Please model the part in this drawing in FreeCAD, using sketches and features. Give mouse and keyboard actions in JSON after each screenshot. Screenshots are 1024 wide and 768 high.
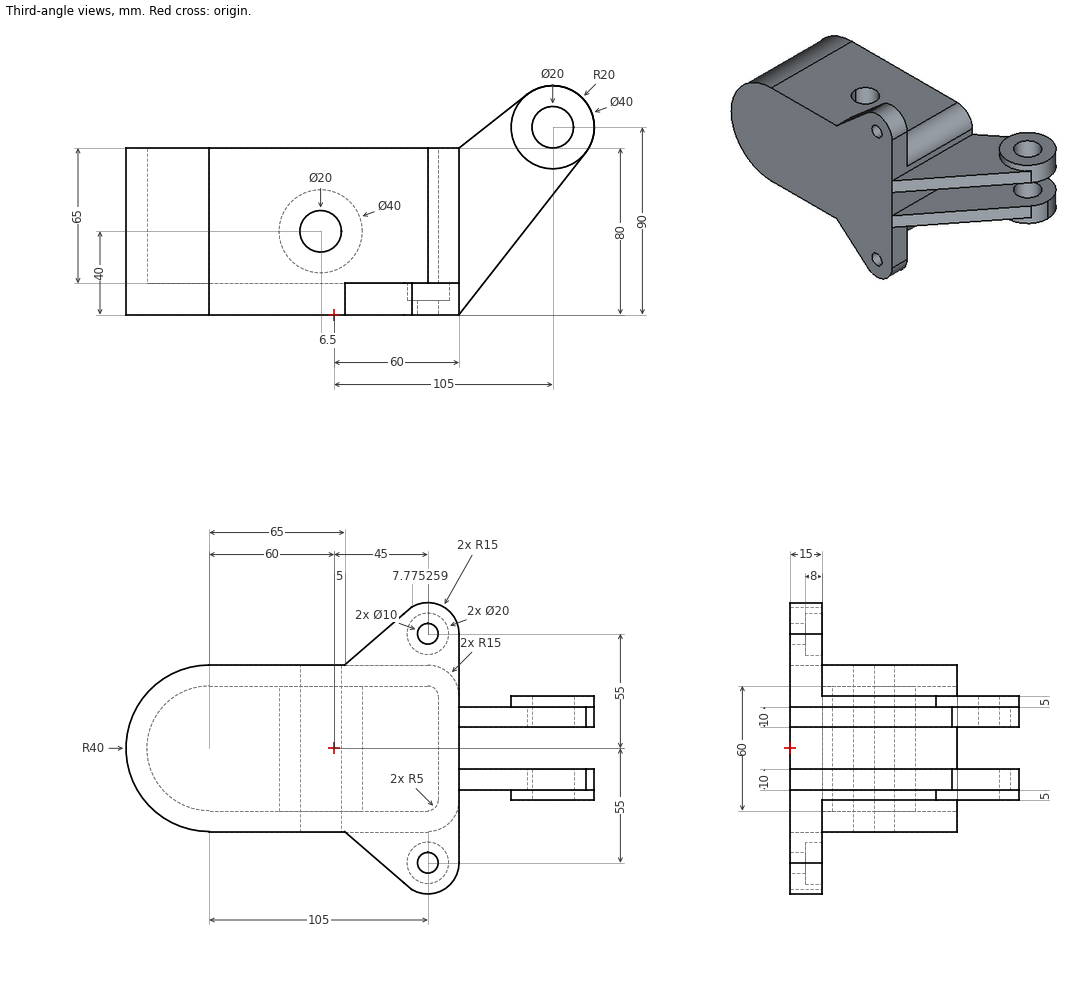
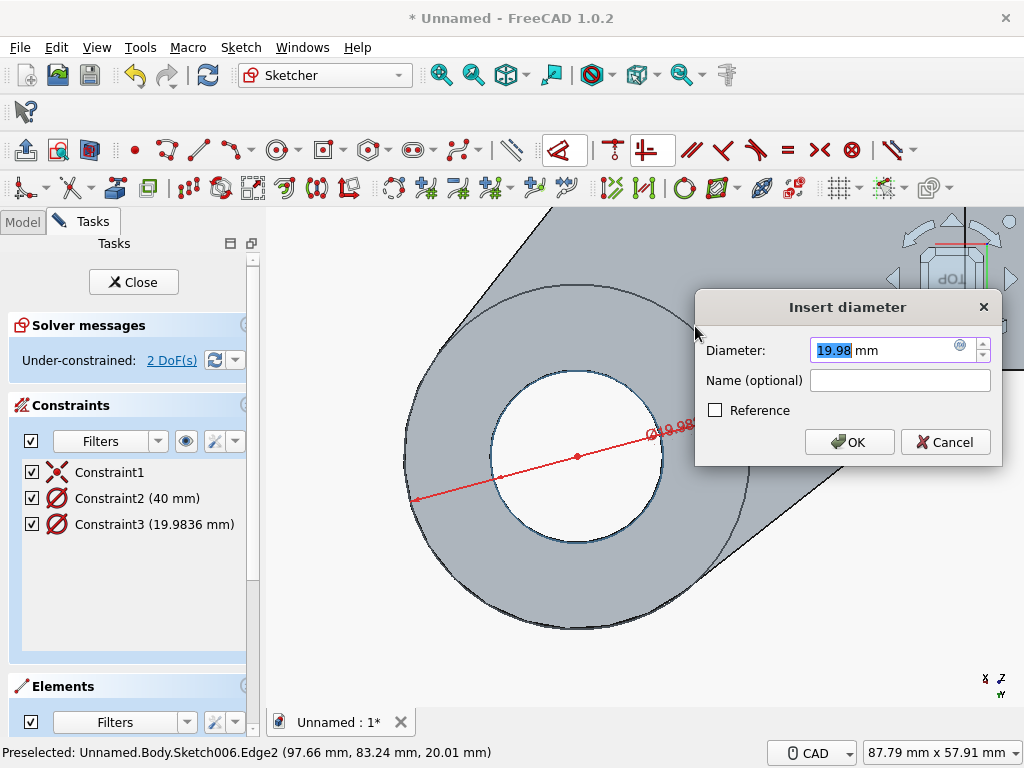
{"action": "type", "text": "20"}
{"action": "key", "text": "Return"}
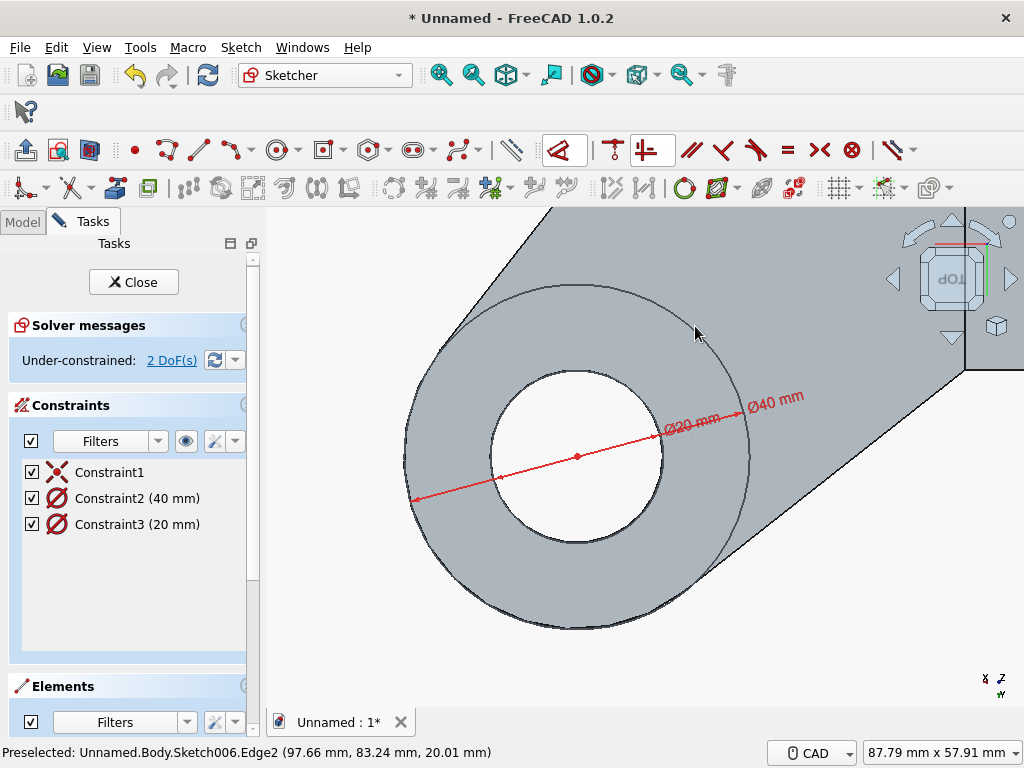
{"action": "left_click", "coordinate": [577, 457]}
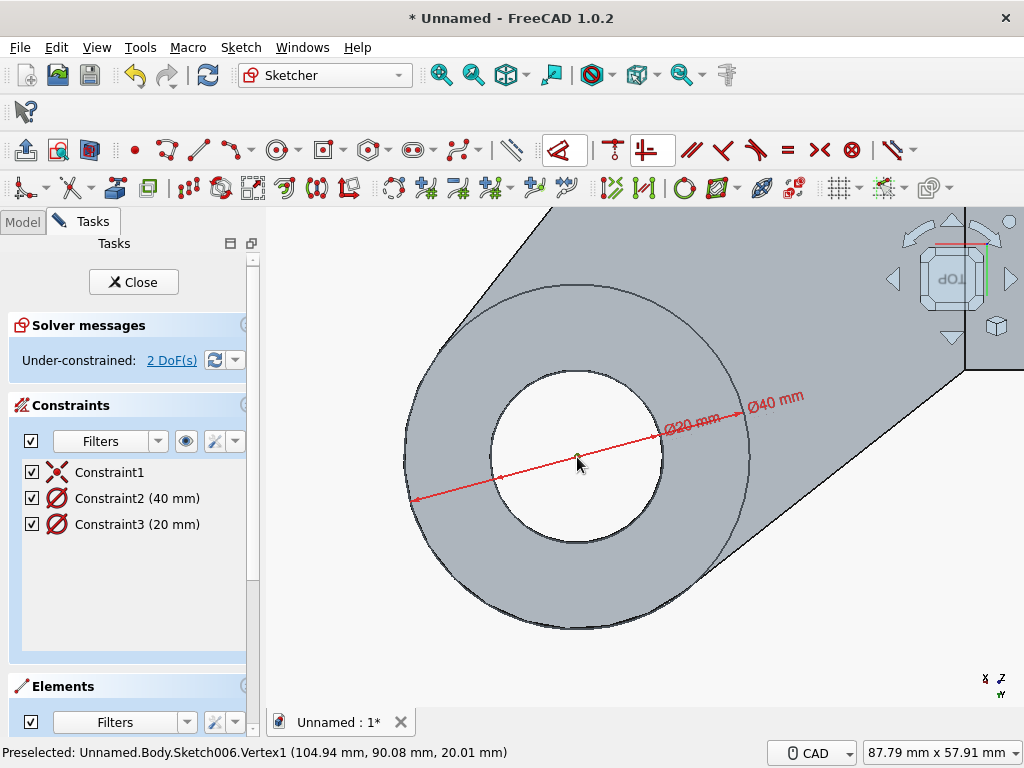
{"action": "left_click", "coordinate": [582, 150]}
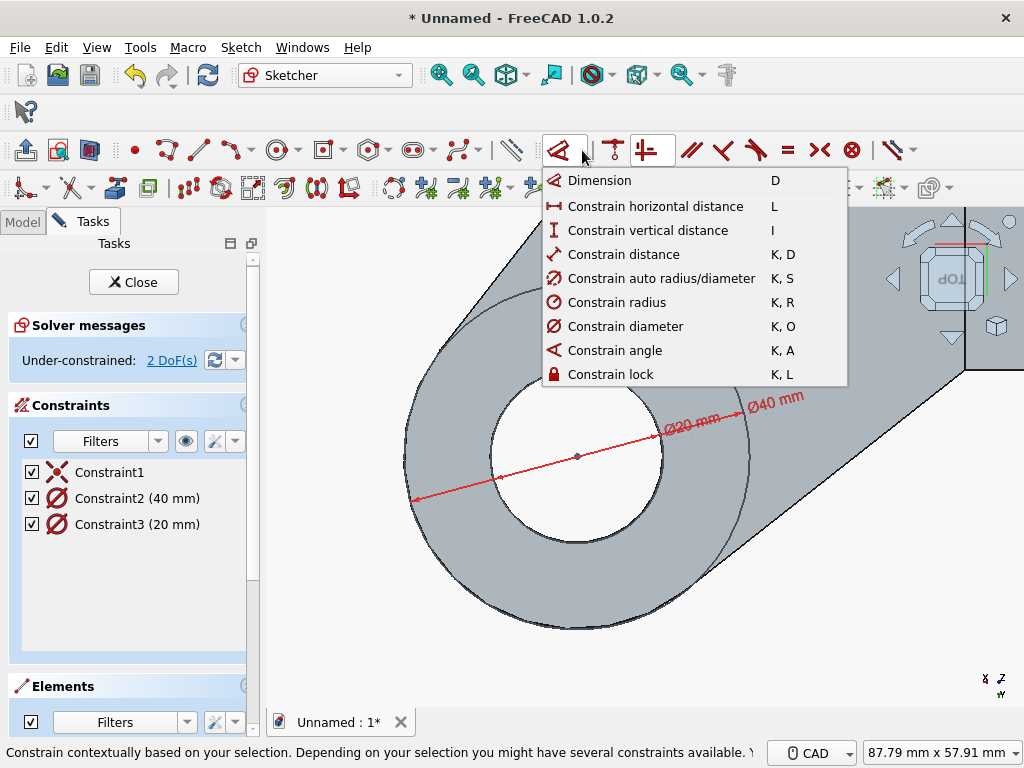
{"action": "left_click", "coordinate": [695, 230]}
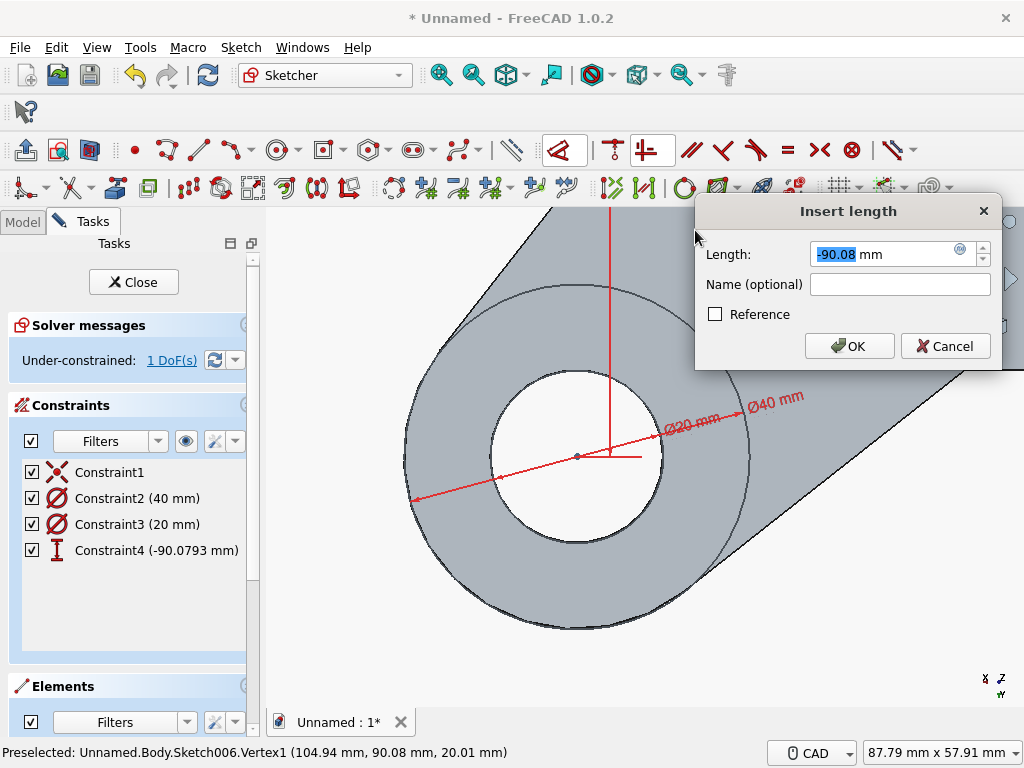
{"action": "type", "text": "-90"}
{"action": "key", "text": "Return"}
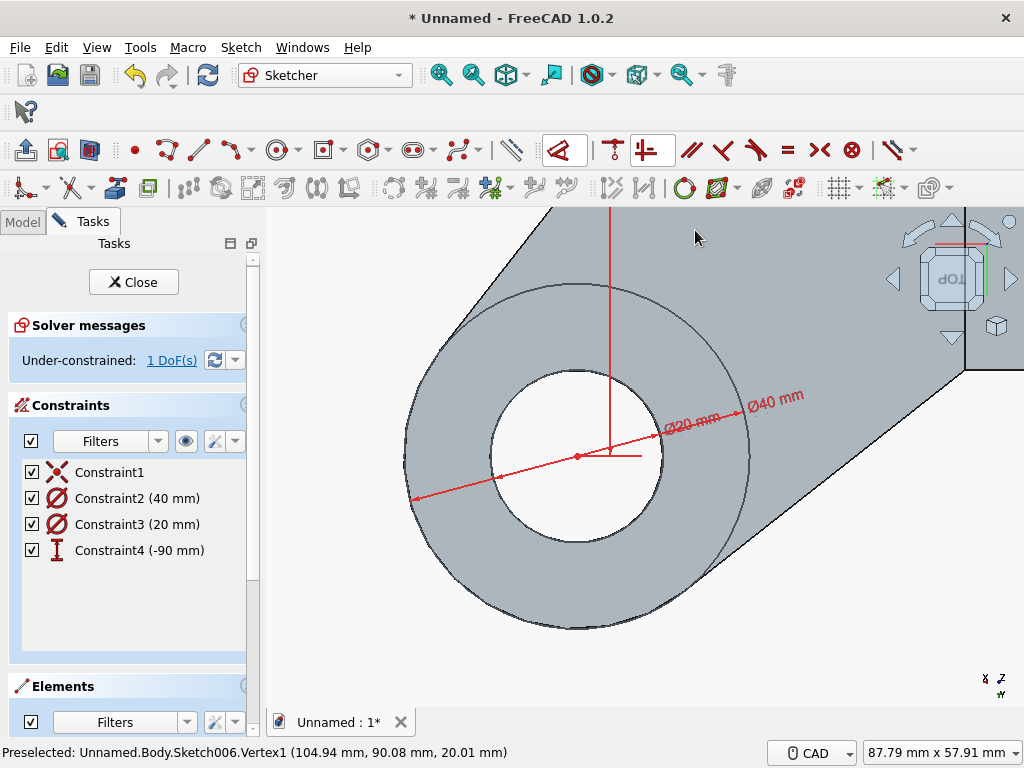
{"action": "left_click", "coordinate": [577, 456]}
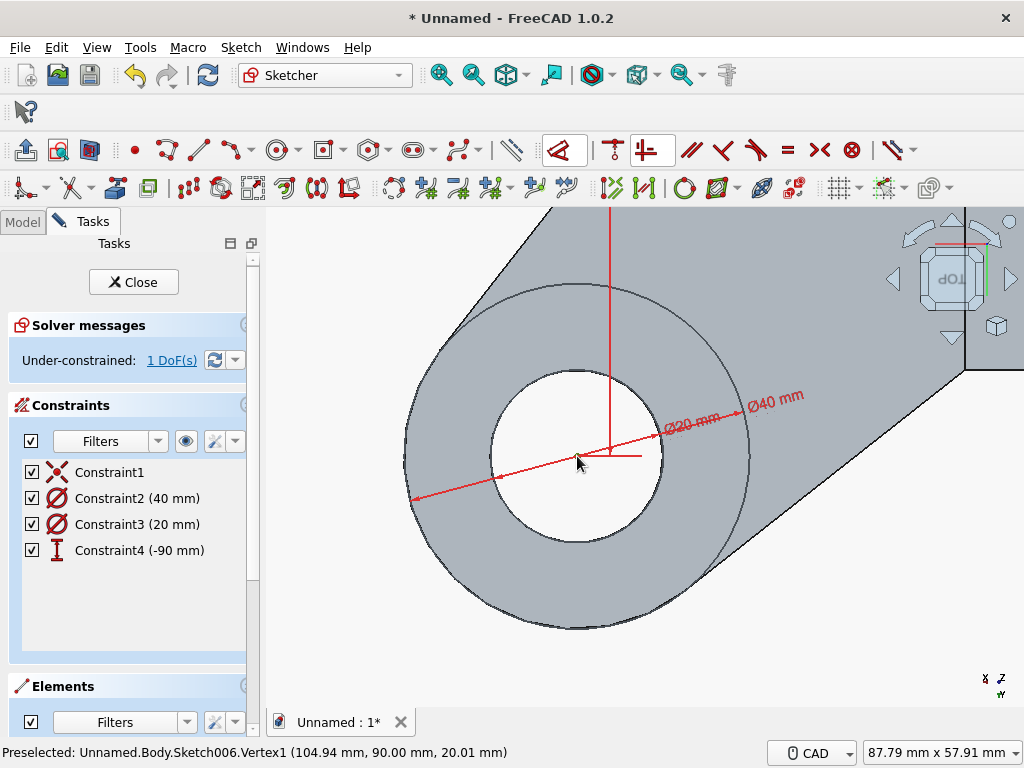
{"action": "left_click", "coordinate": [582, 150]}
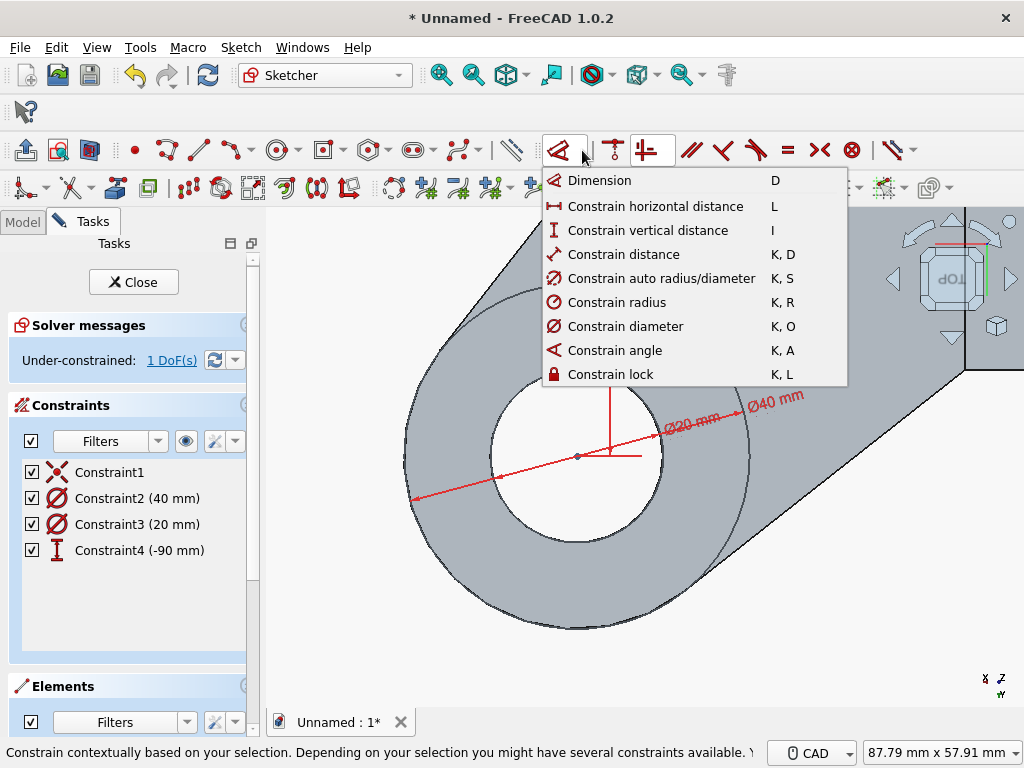
{"action": "left_click", "coordinate": [695, 206]}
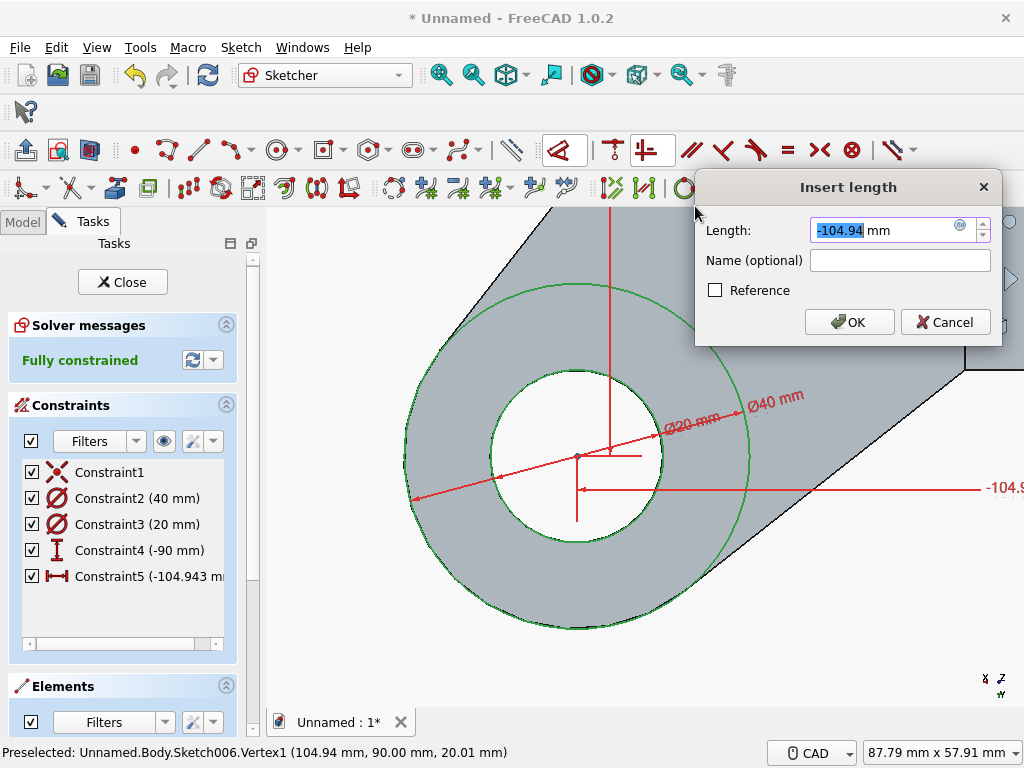
{"action": "type", "text": "-105"}
{"action": "key", "text": "Return"}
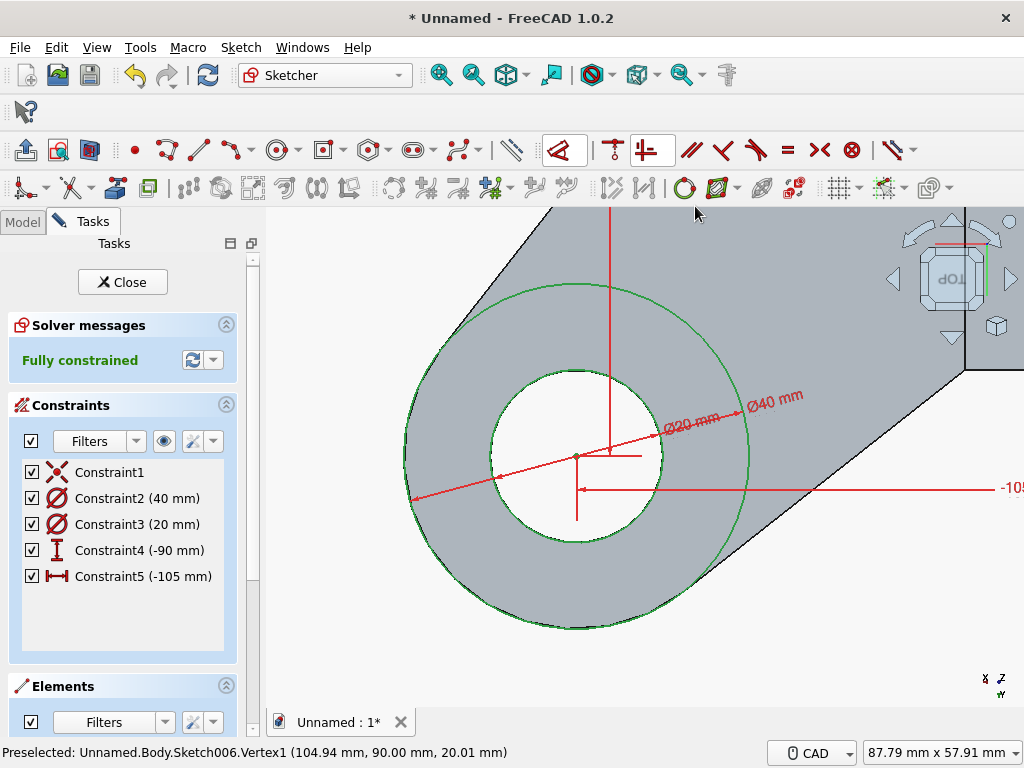
{"action": "left_click", "coordinate": [123, 282]}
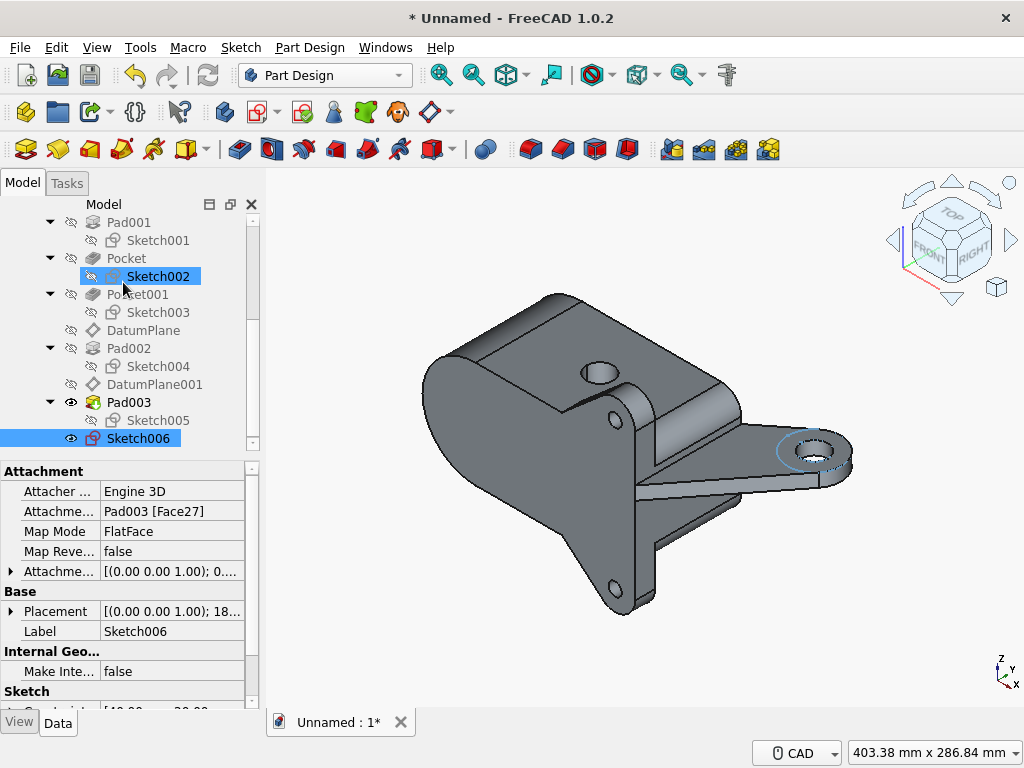
{"action": "left_click", "coordinate": [26, 150]}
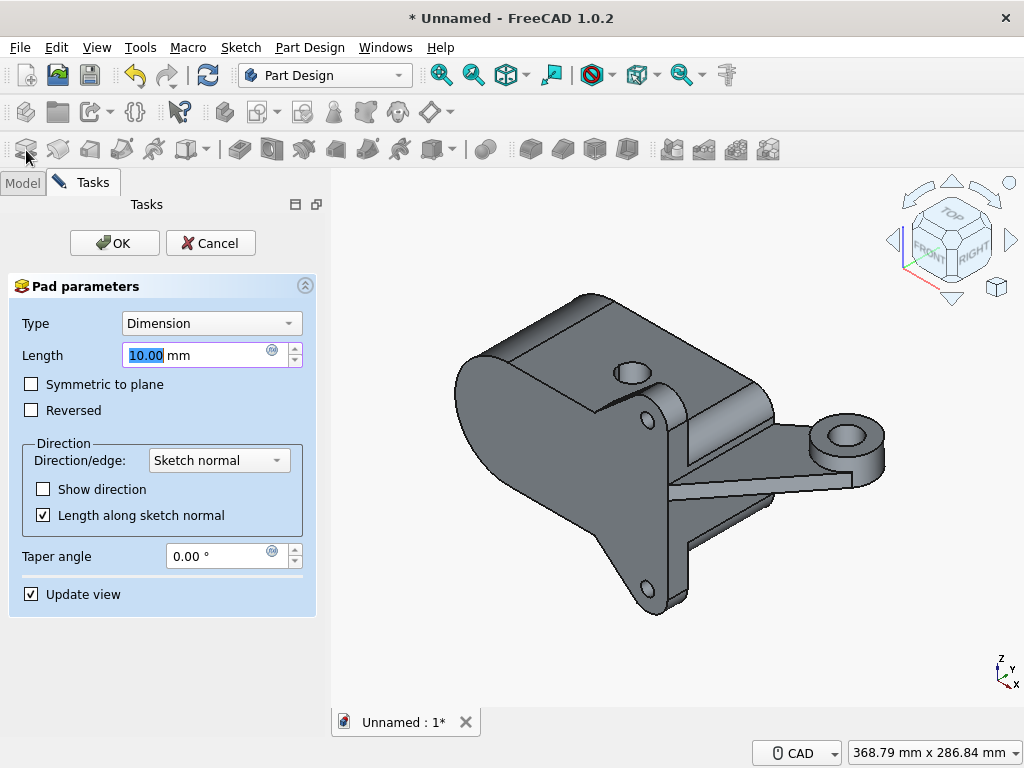
{"action": "type", "text": "5"}
{"action": "key", "text": "Tab"}